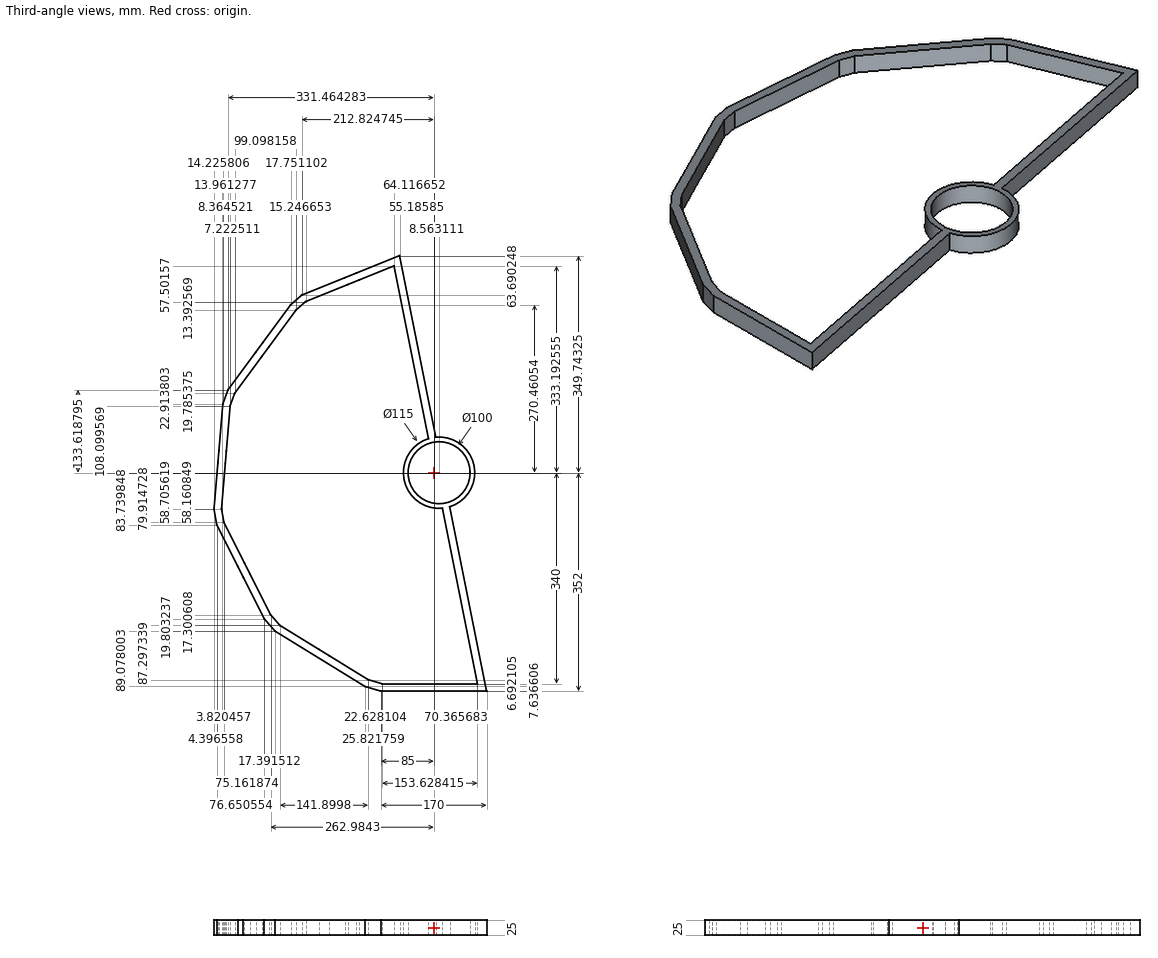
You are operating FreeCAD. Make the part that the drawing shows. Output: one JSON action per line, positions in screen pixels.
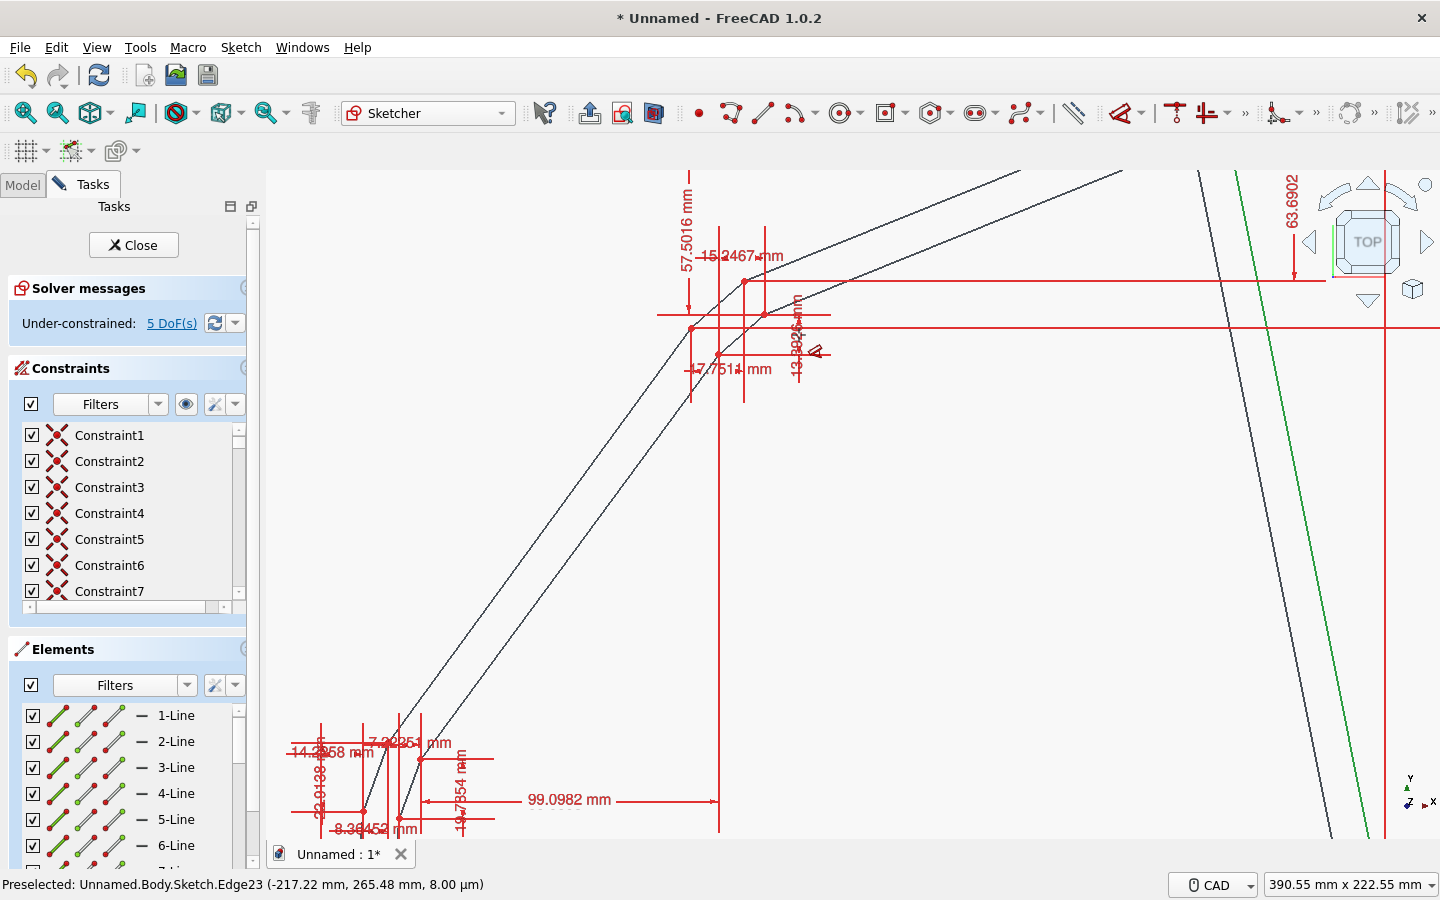
{"action": "scroll", "coordinate": [735, 343], "scroll_direction": "down", "scroll_amount": 8}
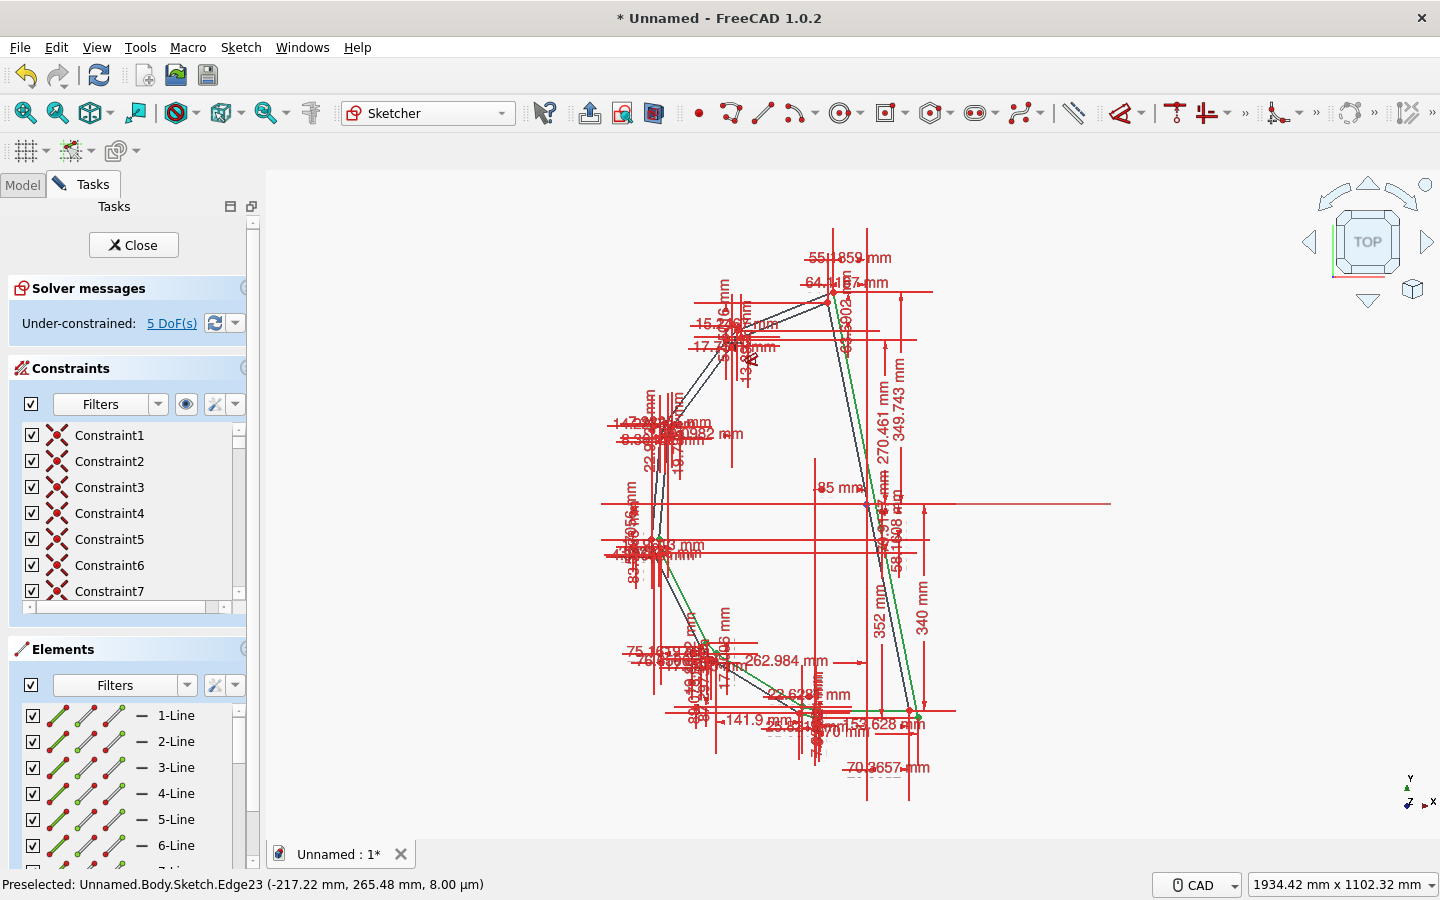
{"action": "scroll", "coordinate": [737, 331], "scroll_direction": "up", "scroll_amount": 3}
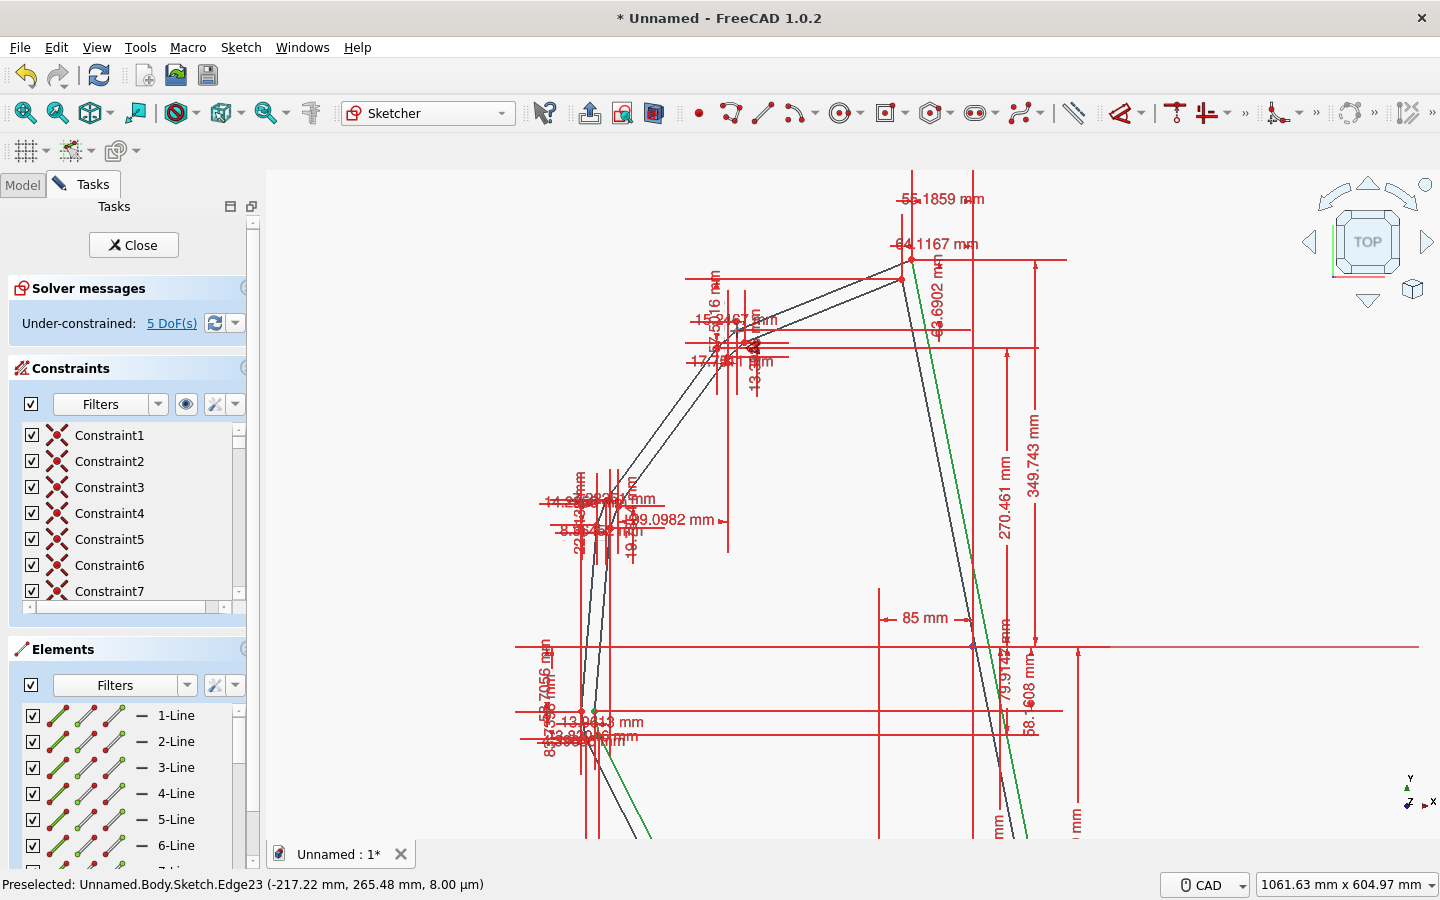
{"action": "left_click", "coordinate": [737, 330]}
{"action": "left_click", "coordinate": [855, 681]}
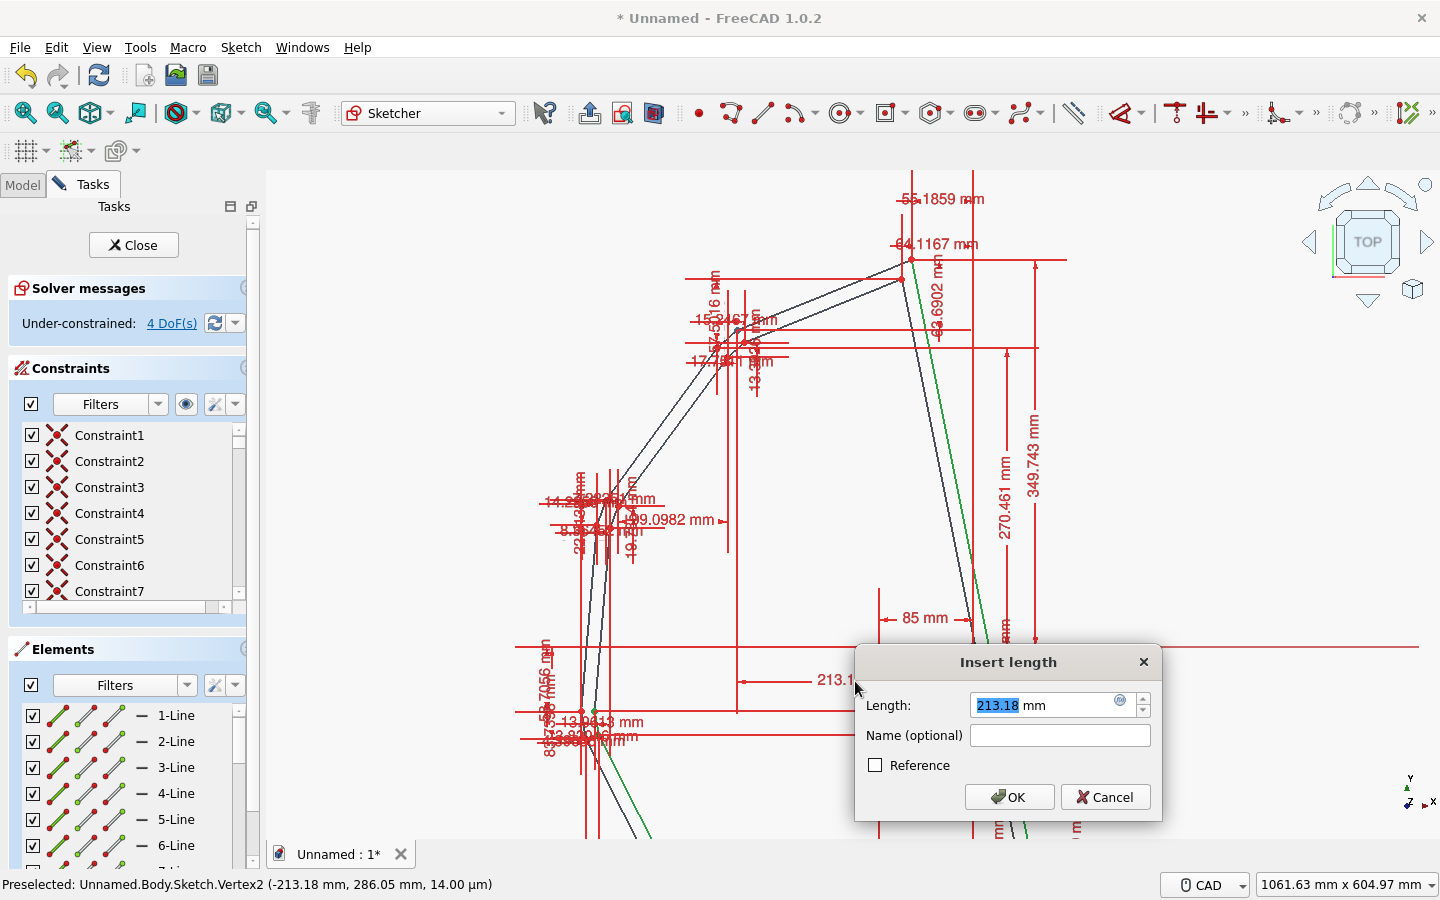
{"action": "type", "text": "212.824745"}
{"action": "key", "text": "Return"}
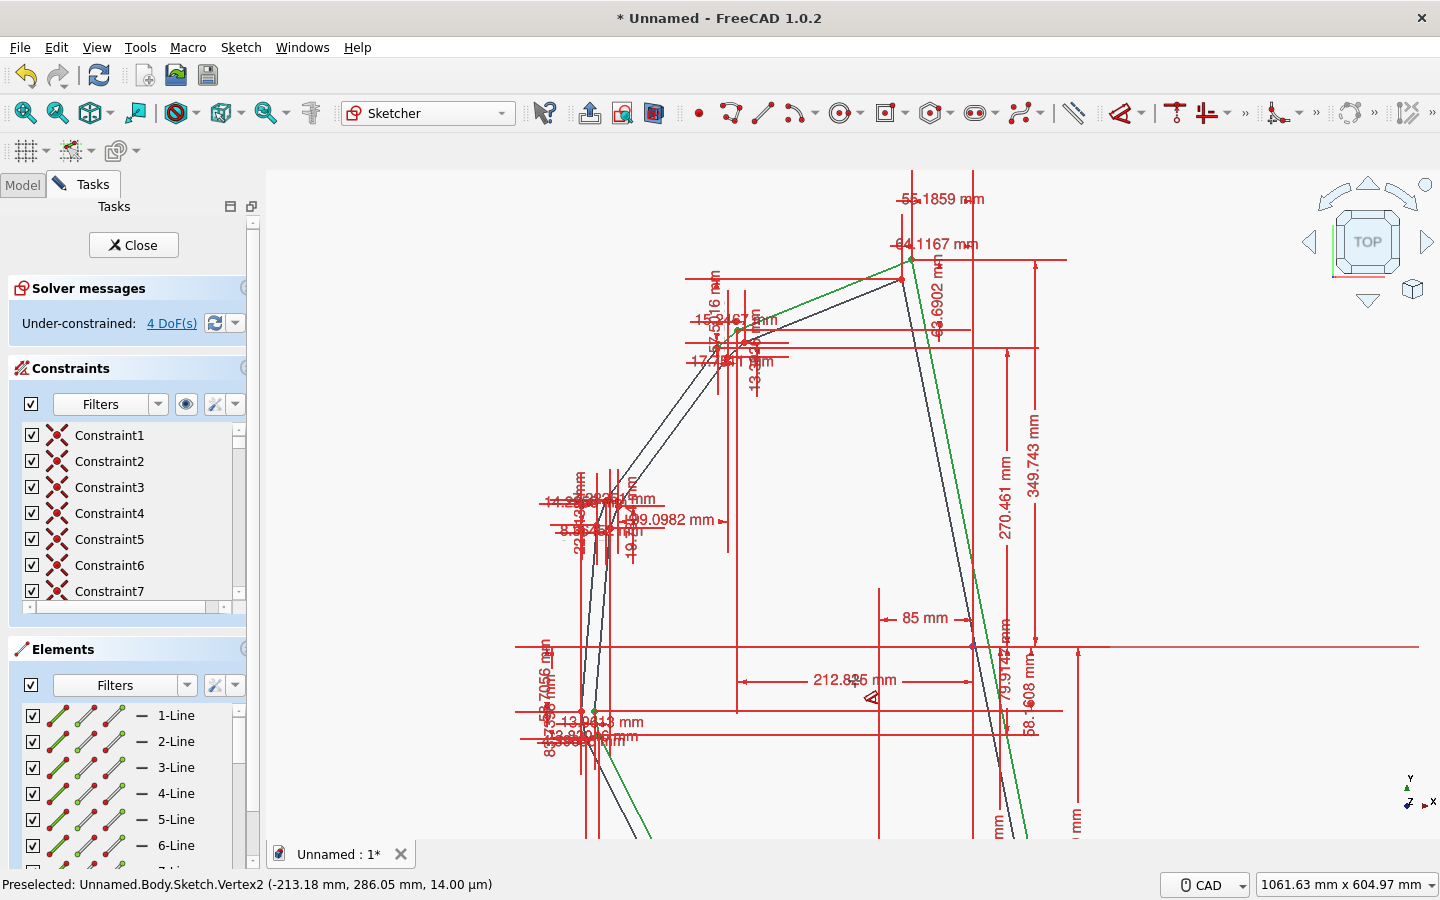
{"action": "left_click", "coordinate": [606, 500]}
{"action": "left_click", "coordinate": [789, 466]}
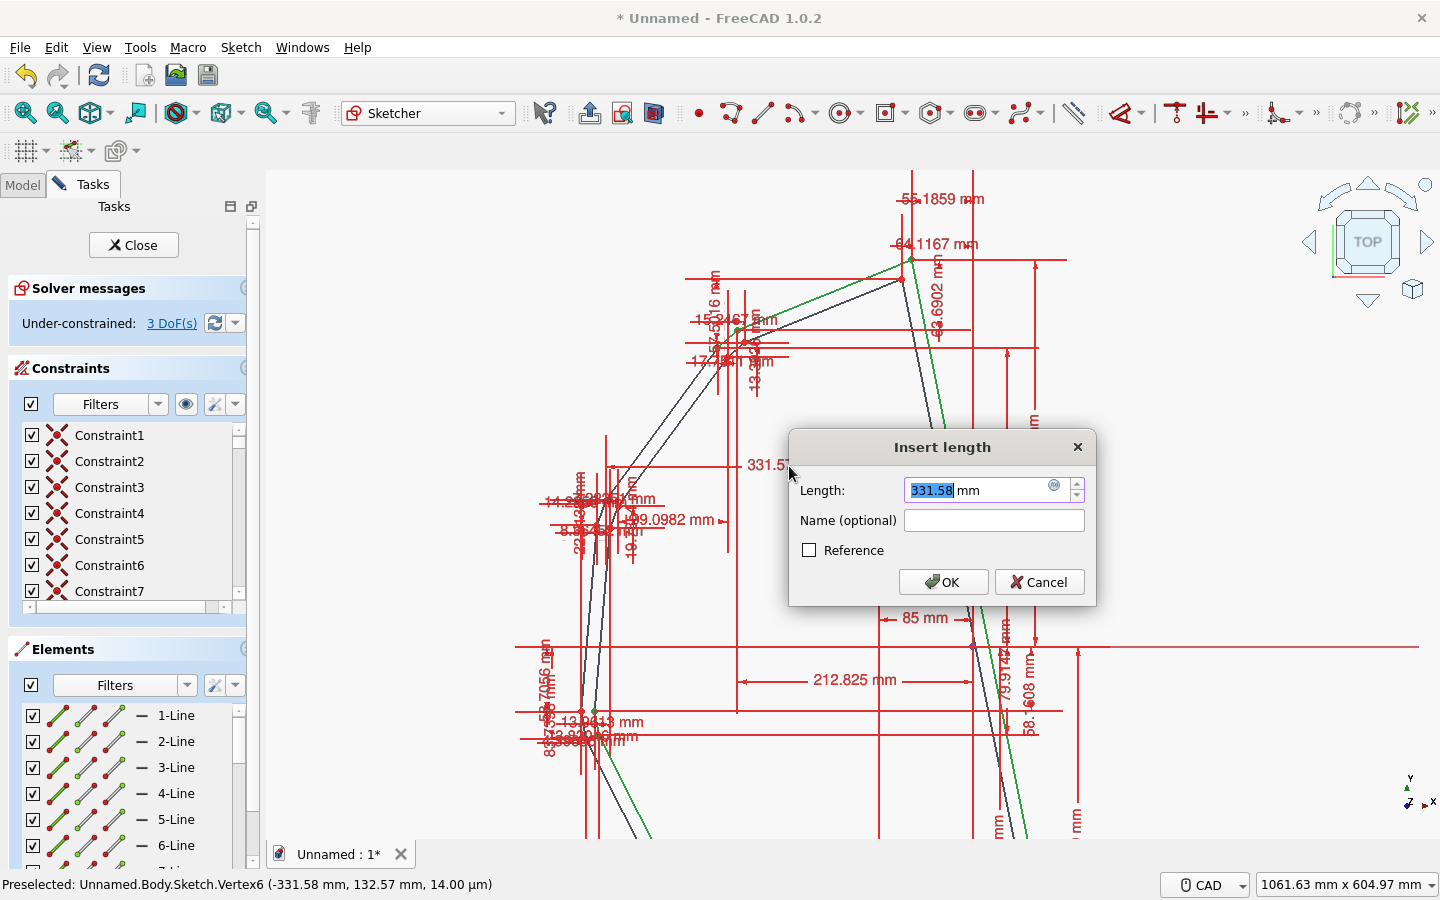
{"action": "type", "text": "331.464283"}
{"action": "key", "text": "Return"}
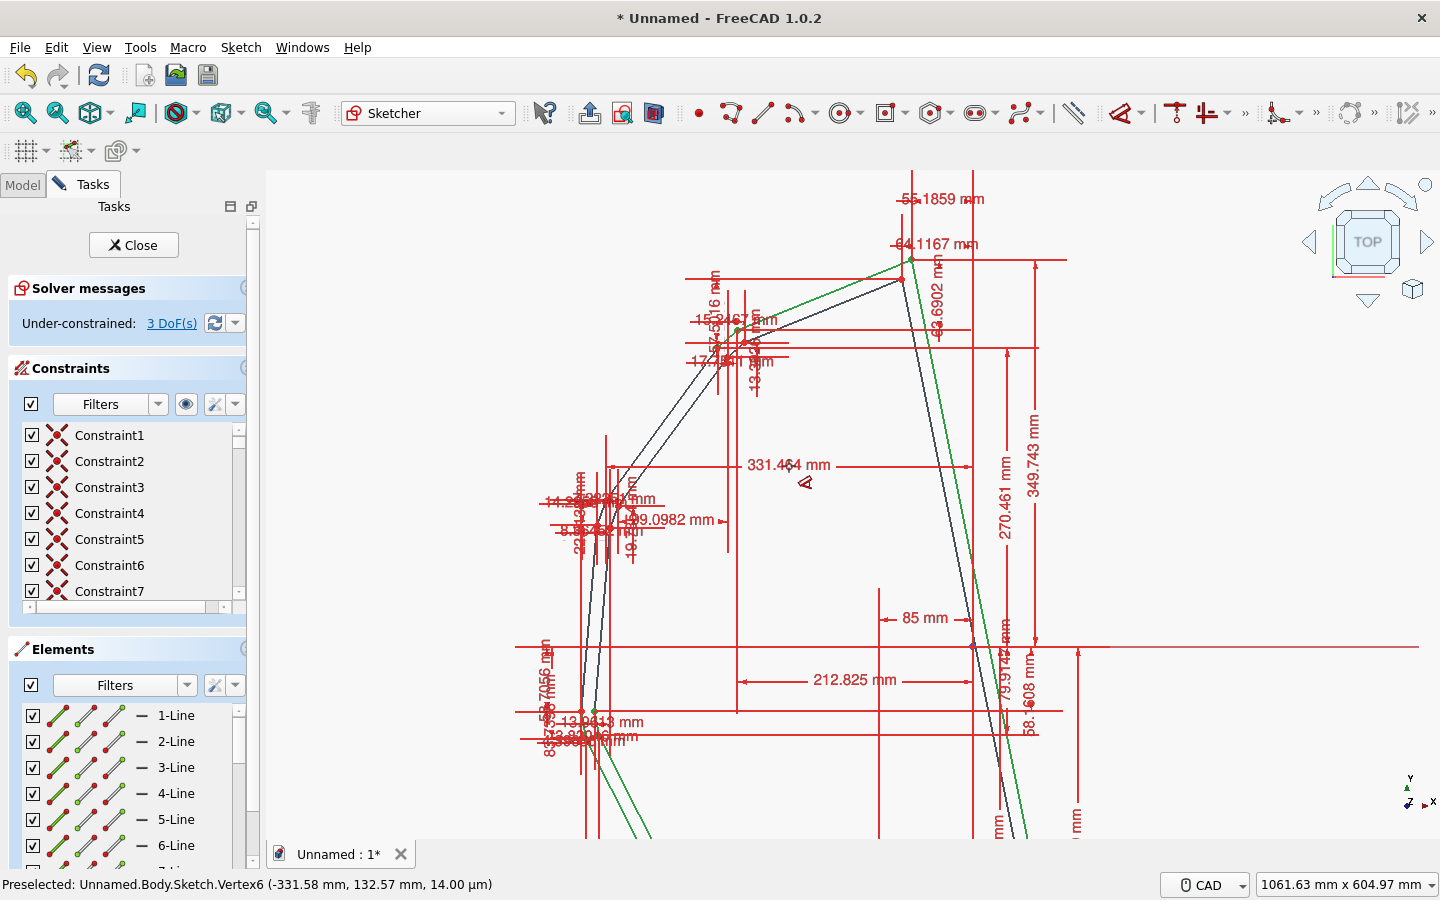
{"action": "left_click", "coordinate": [606, 500]}
{"action": "left_click", "coordinate": [572, 573]}